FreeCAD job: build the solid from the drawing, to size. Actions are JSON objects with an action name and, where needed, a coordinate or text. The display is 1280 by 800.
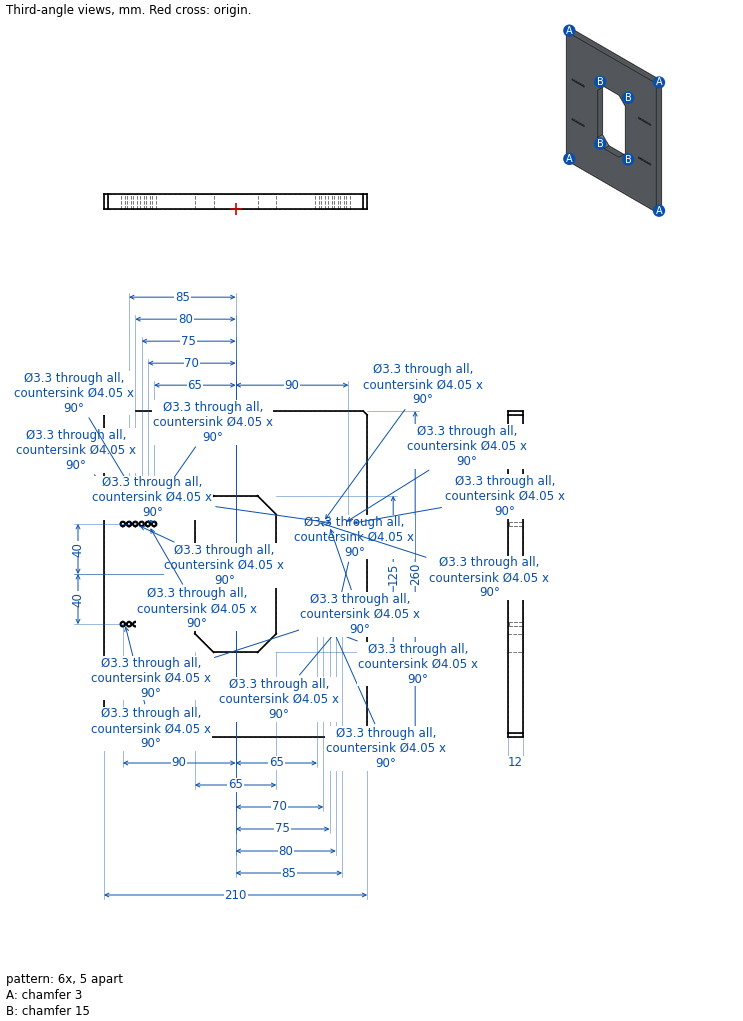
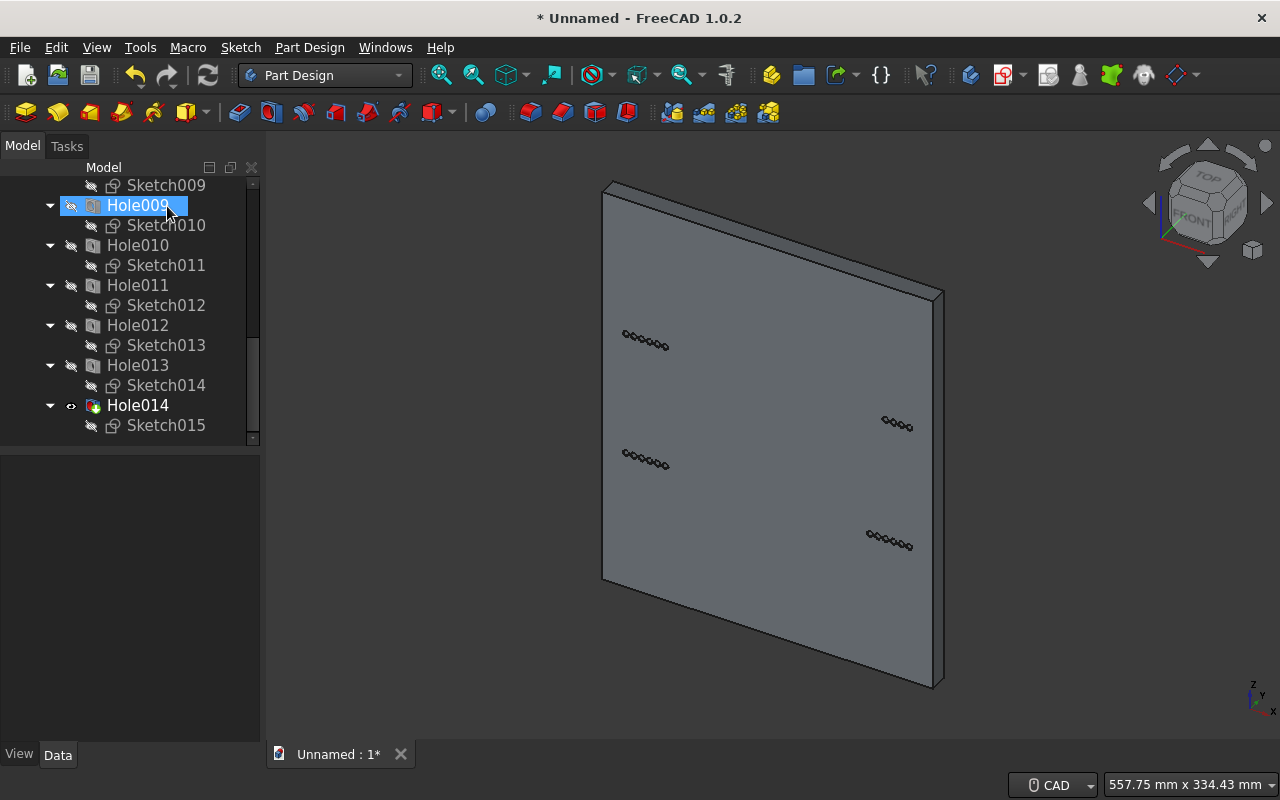
{"action": "left_click", "coordinate": [1004, 76]}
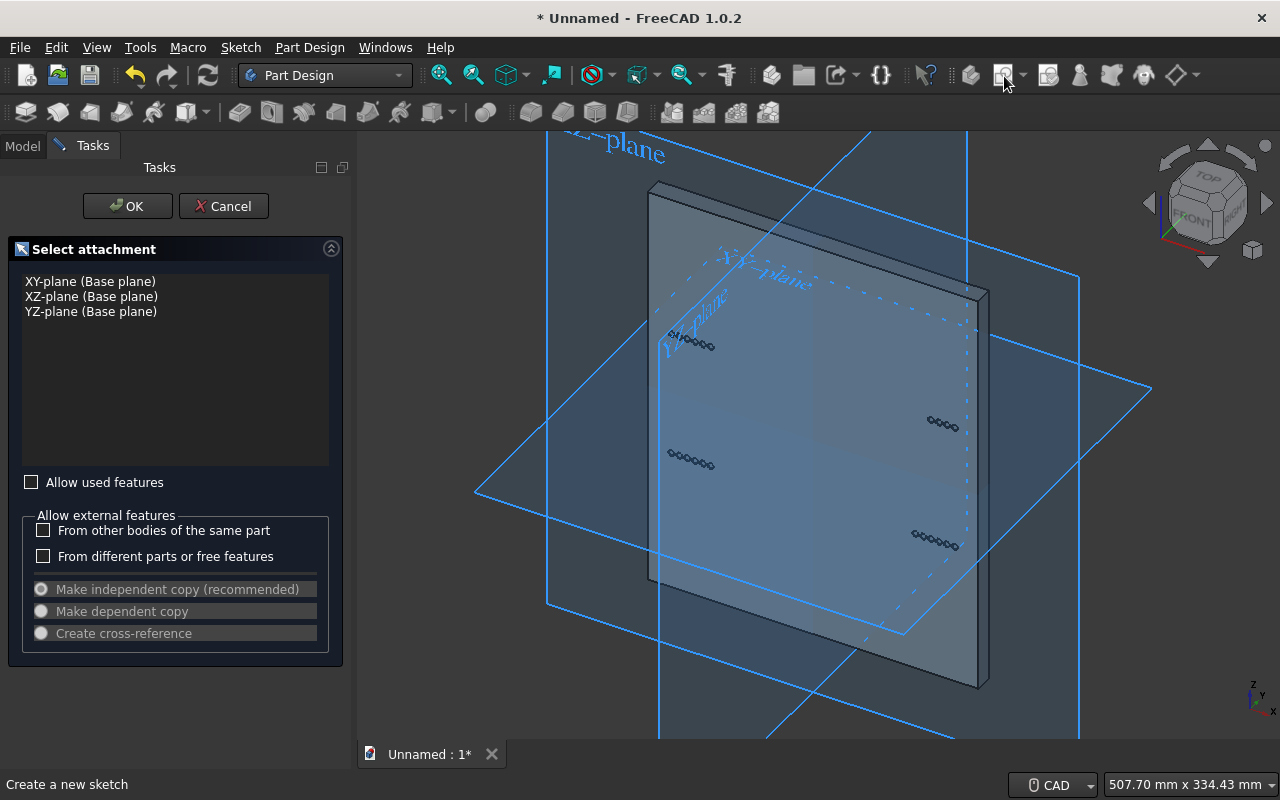
{"action": "left_click", "coordinate": [82, 296]}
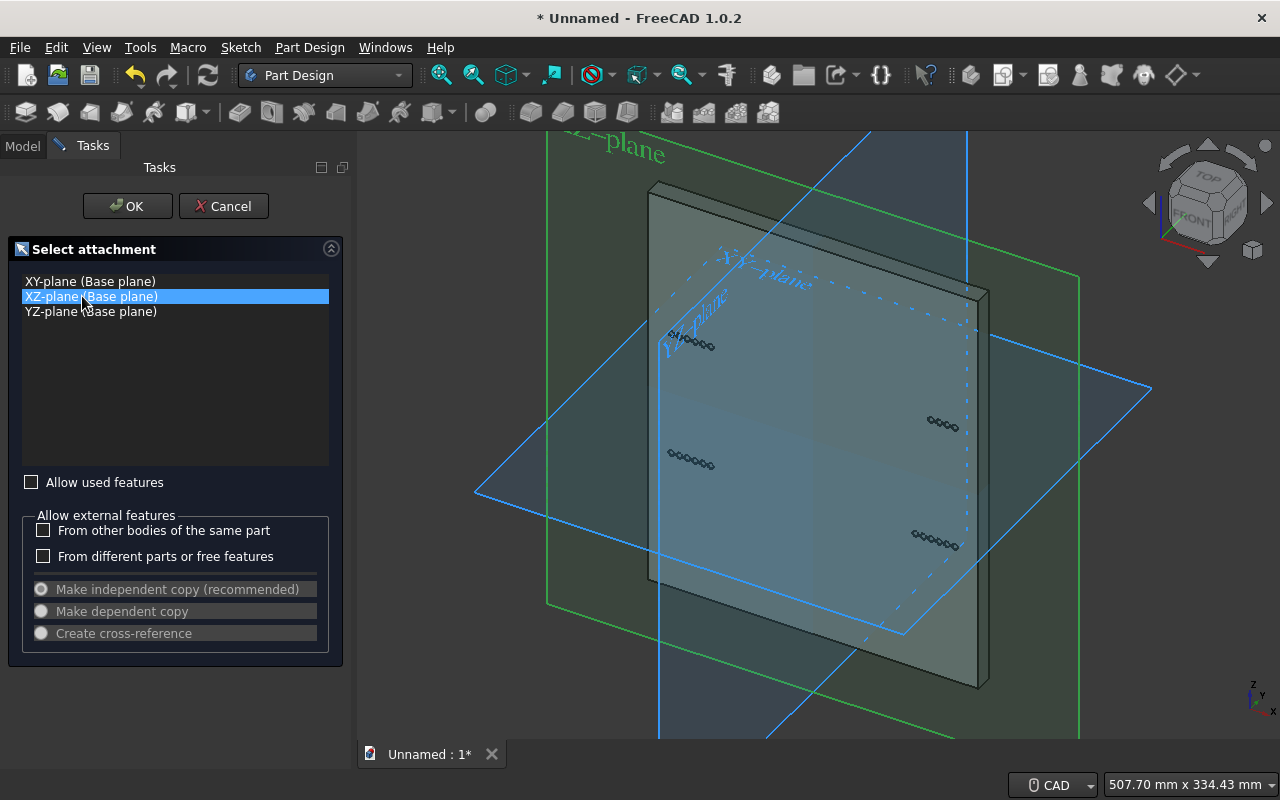
{"action": "left_click", "coordinate": [128, 206]}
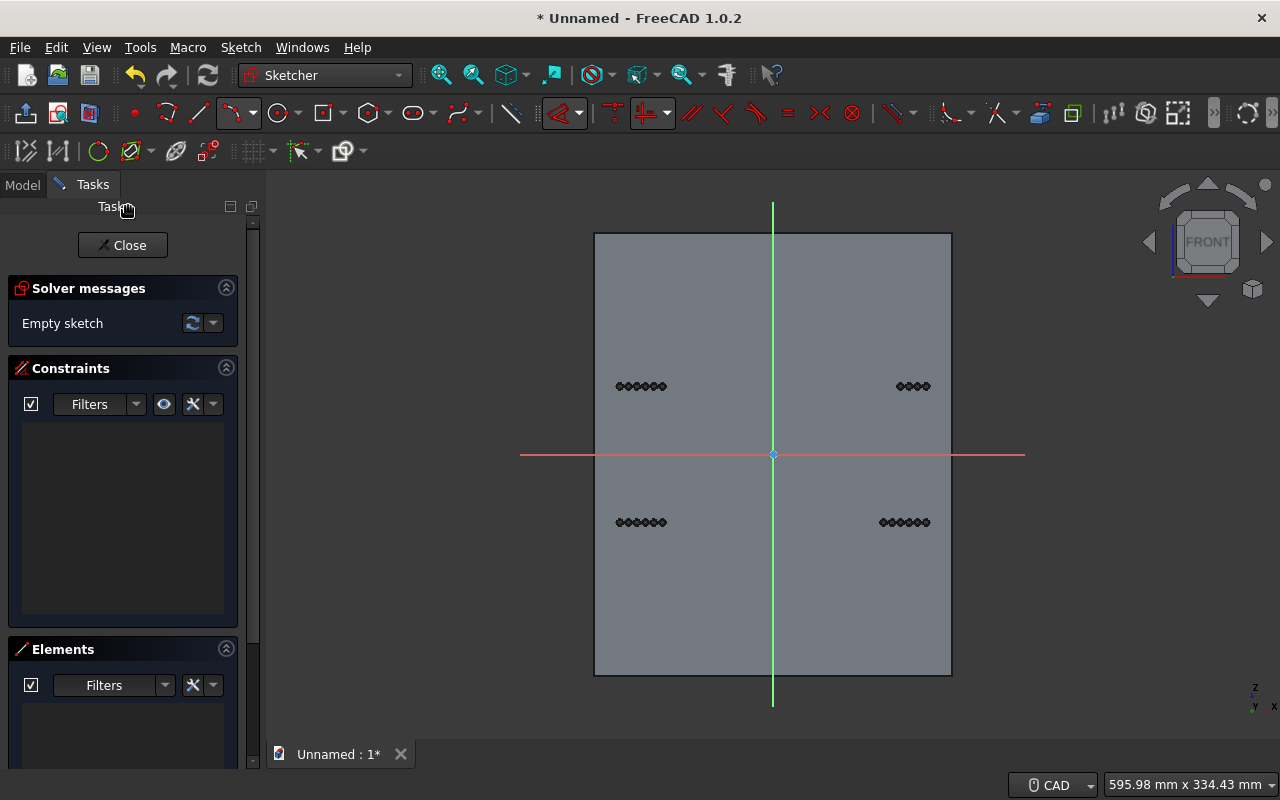
{"action": "scroll", "coordinate": [902, 383], "scroll_direction": "up", "scroll_amount": 15}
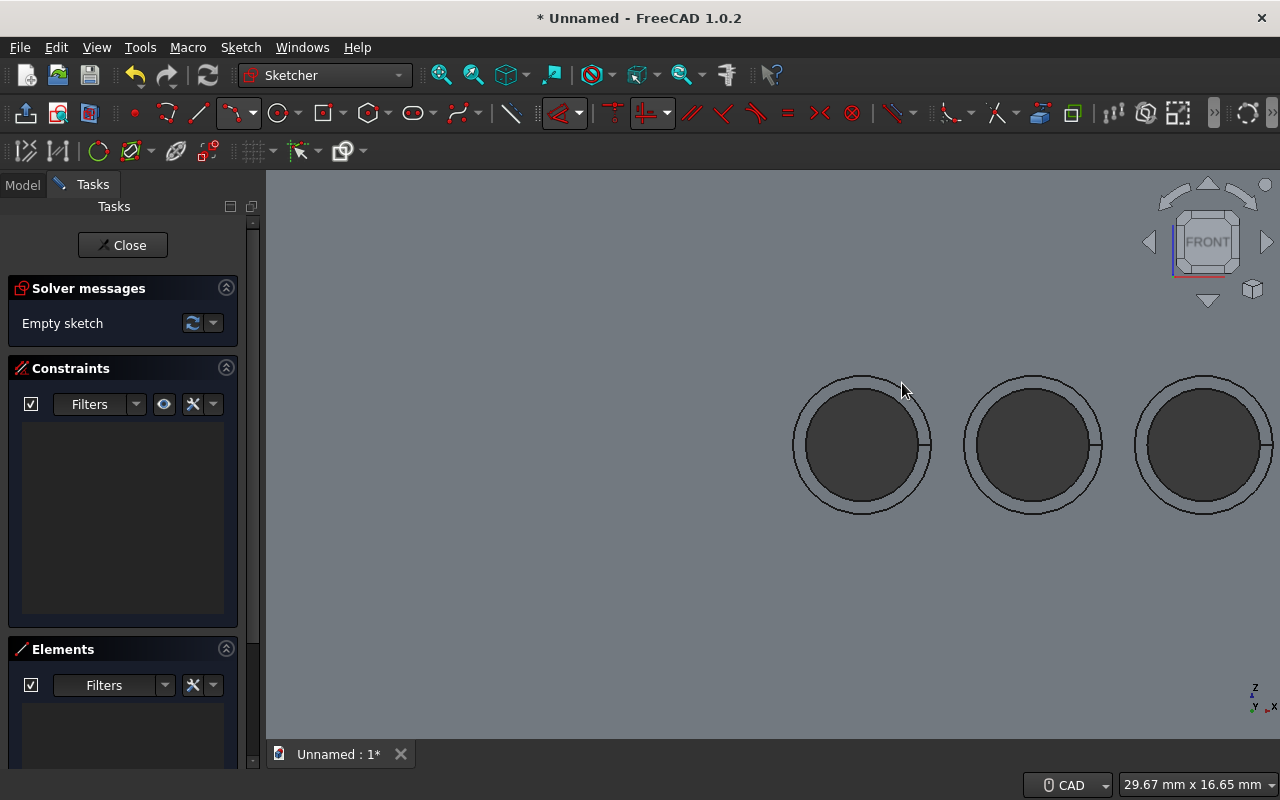
{"action": "scroll", "coordinate": [685, 441], "scroll_direction": "up", "scroll_amount": 6}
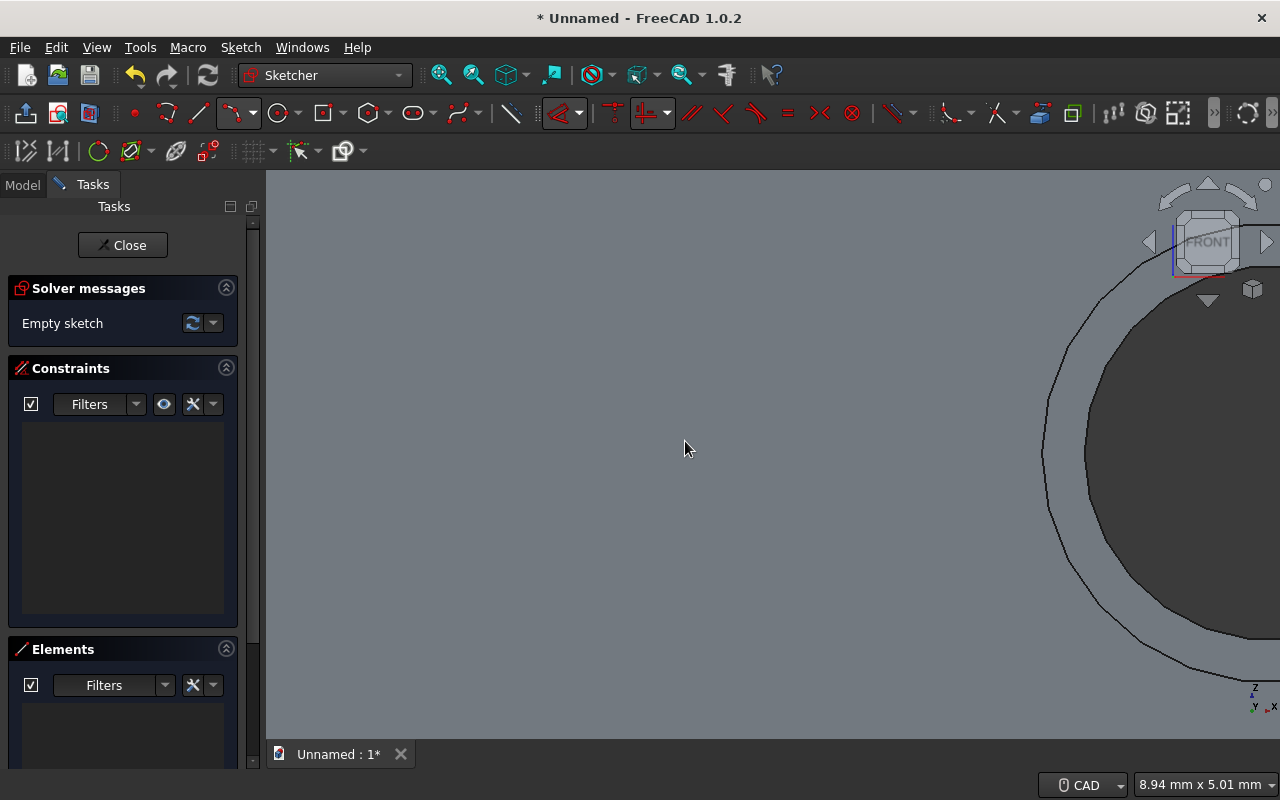
{"action": "left_click", "coordinate": [278, 114]}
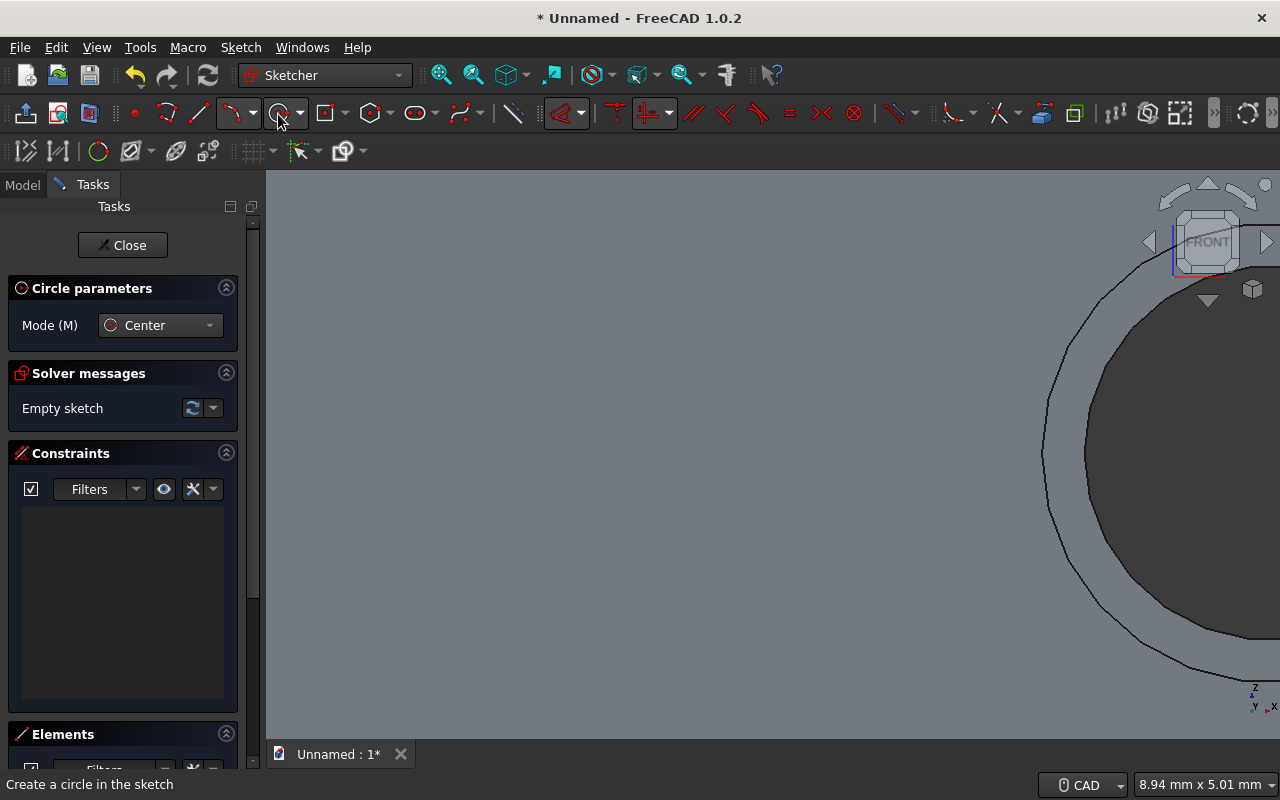
{"action": "left_click", "coordinate": [704, 453]}
{"action": "mouse_move", "coordinate": [837, 321]}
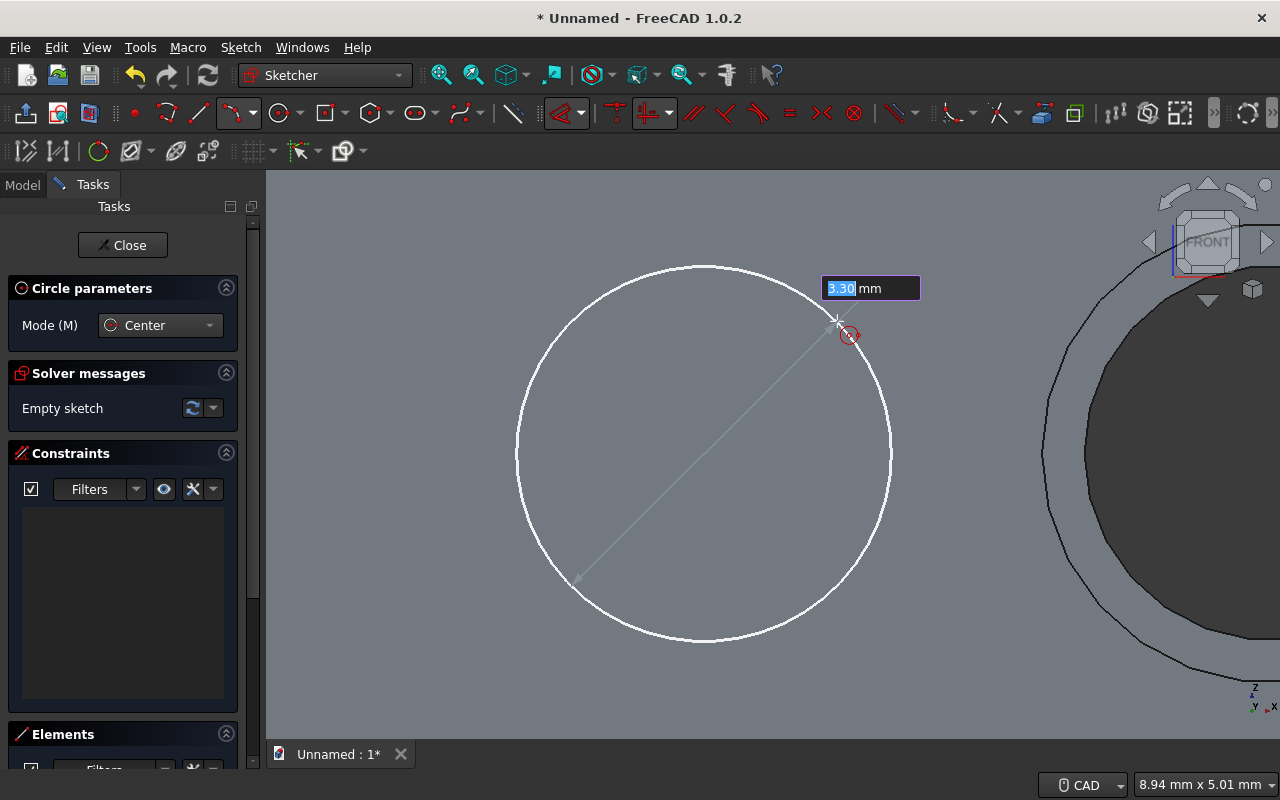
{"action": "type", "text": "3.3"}
{"action": "key", "text": "Return"}
{"action": "key", "text": "Escape"}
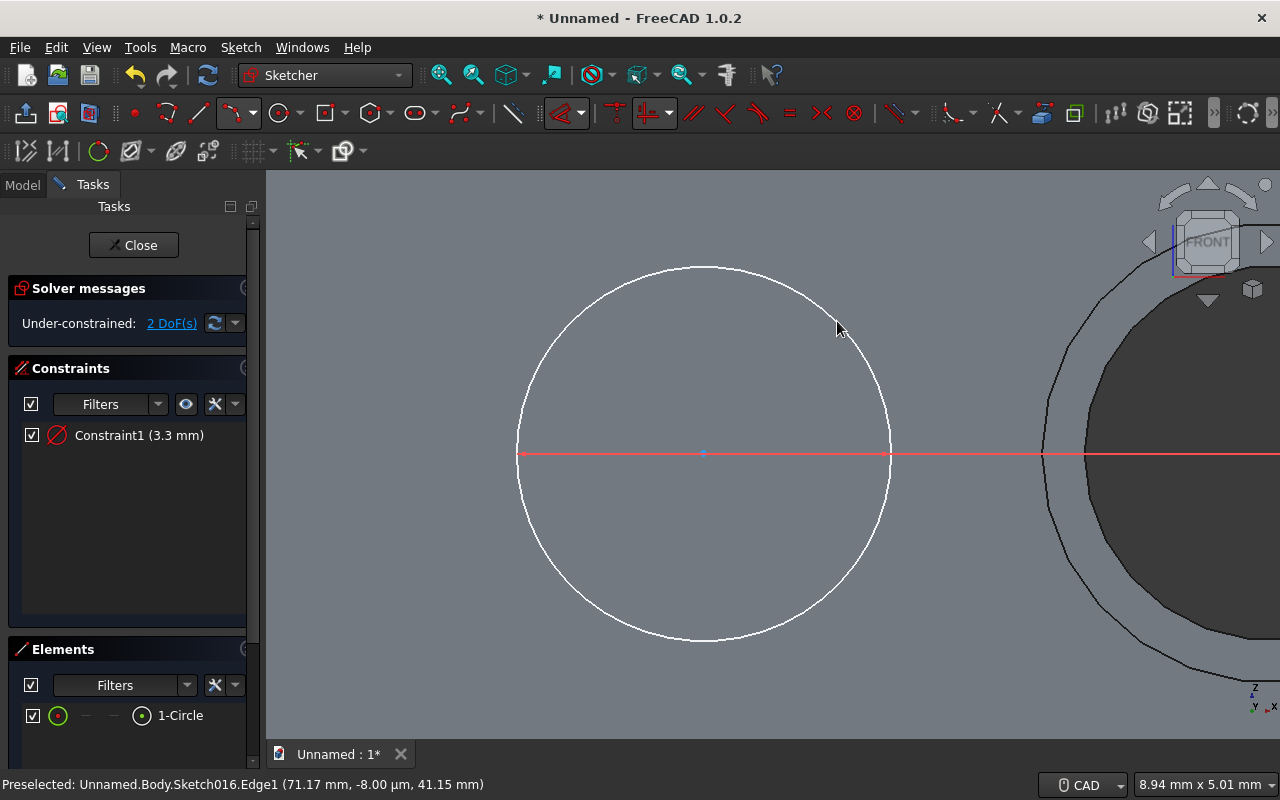
{"action": "left_click", "coordinate": [704, 454]}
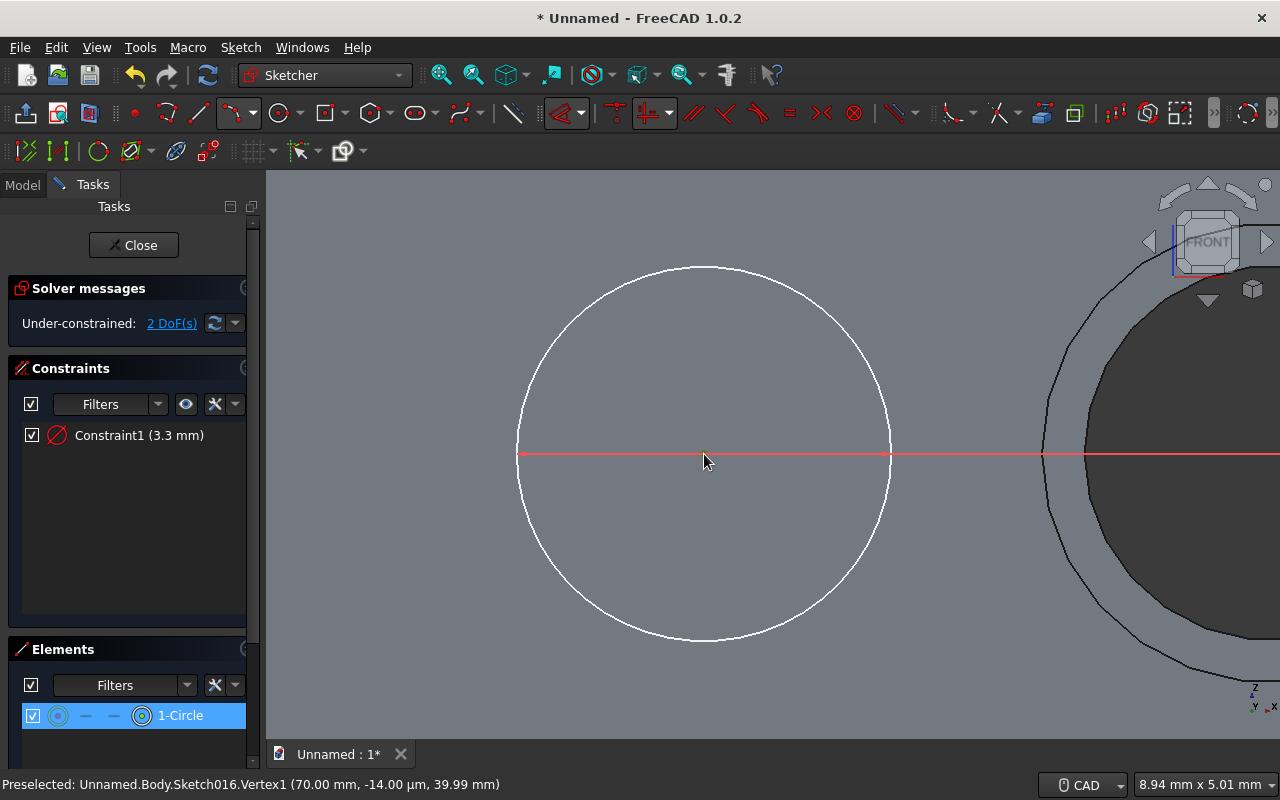
{"action": "left_click", "coordinate": [584, 114]}